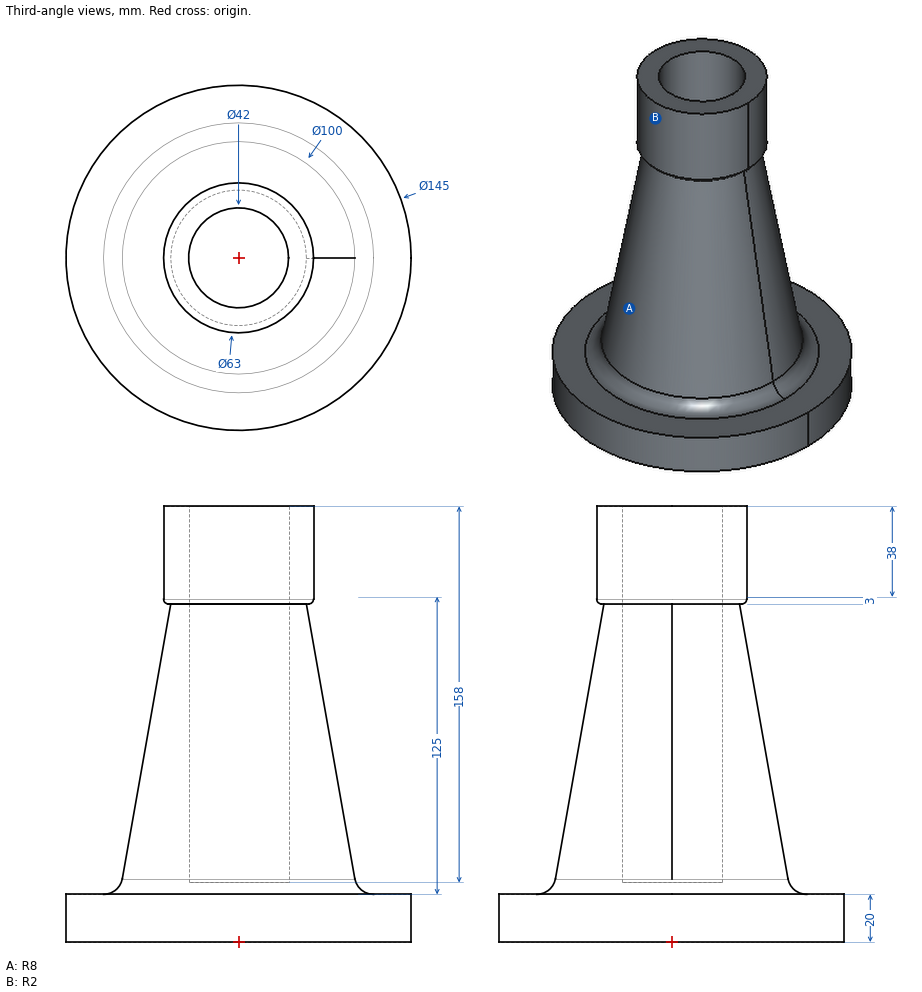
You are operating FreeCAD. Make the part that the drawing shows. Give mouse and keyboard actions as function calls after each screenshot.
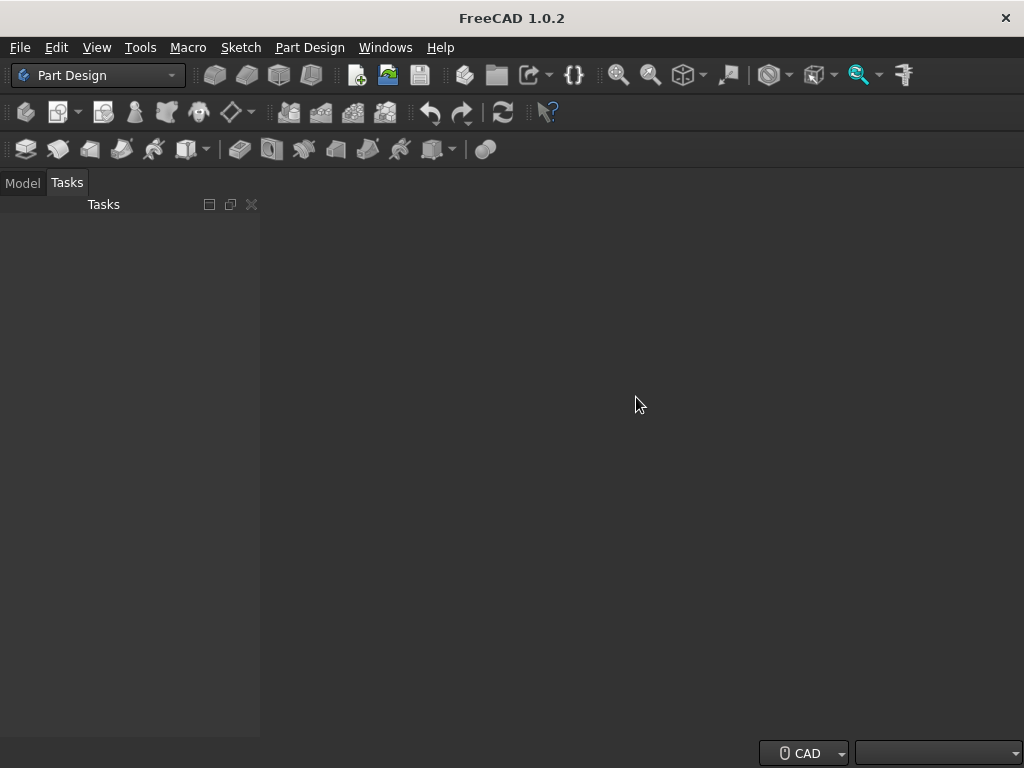
click(356, 76)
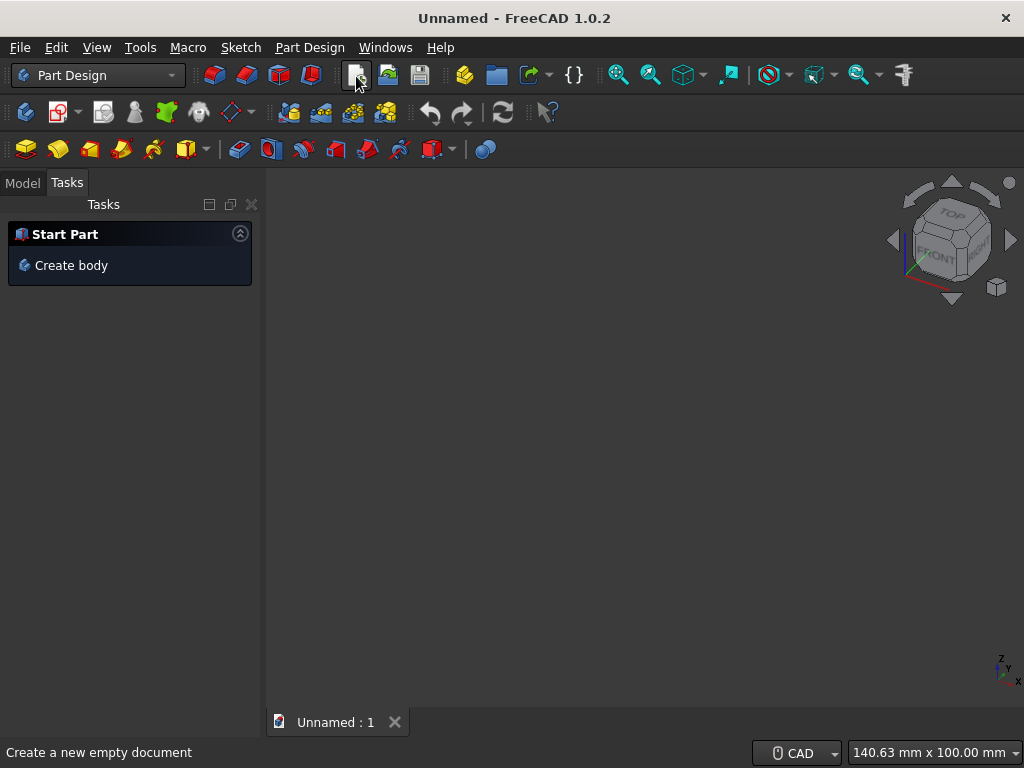
click(58, 112)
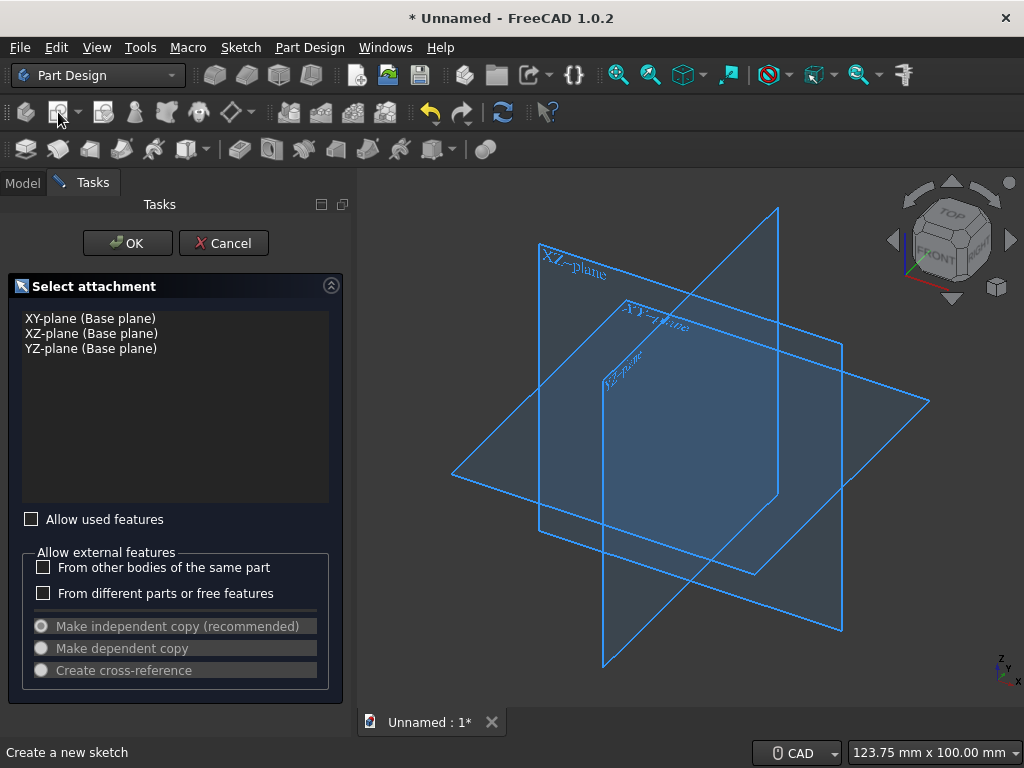
click(82, 318)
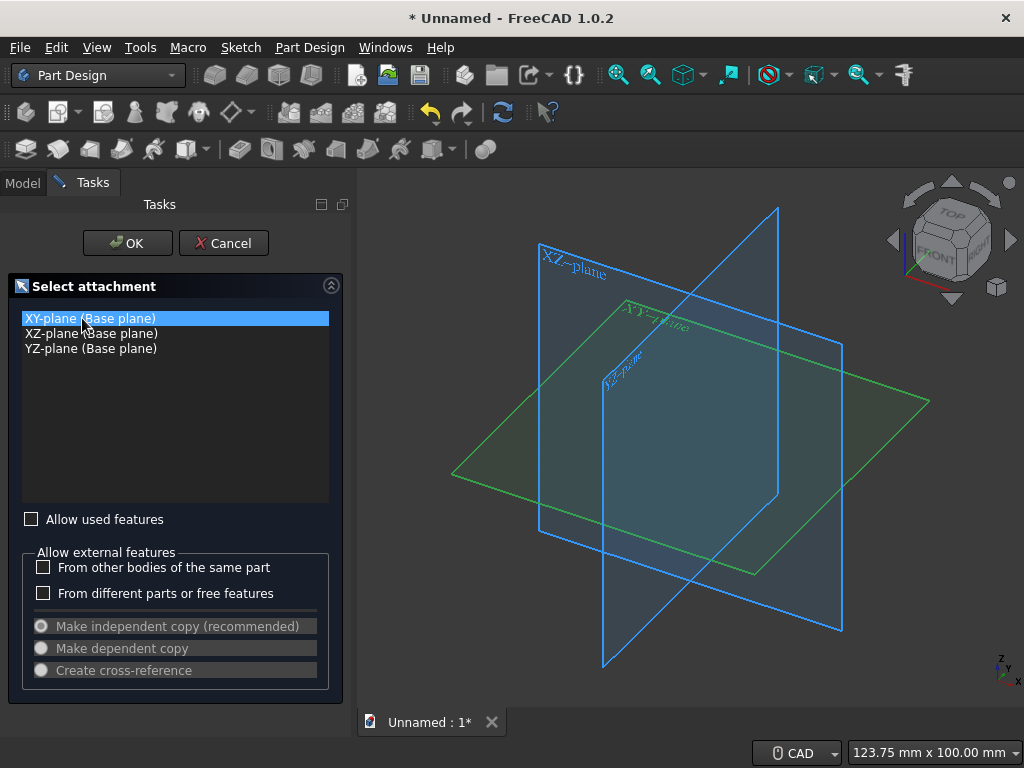
click(128, 243)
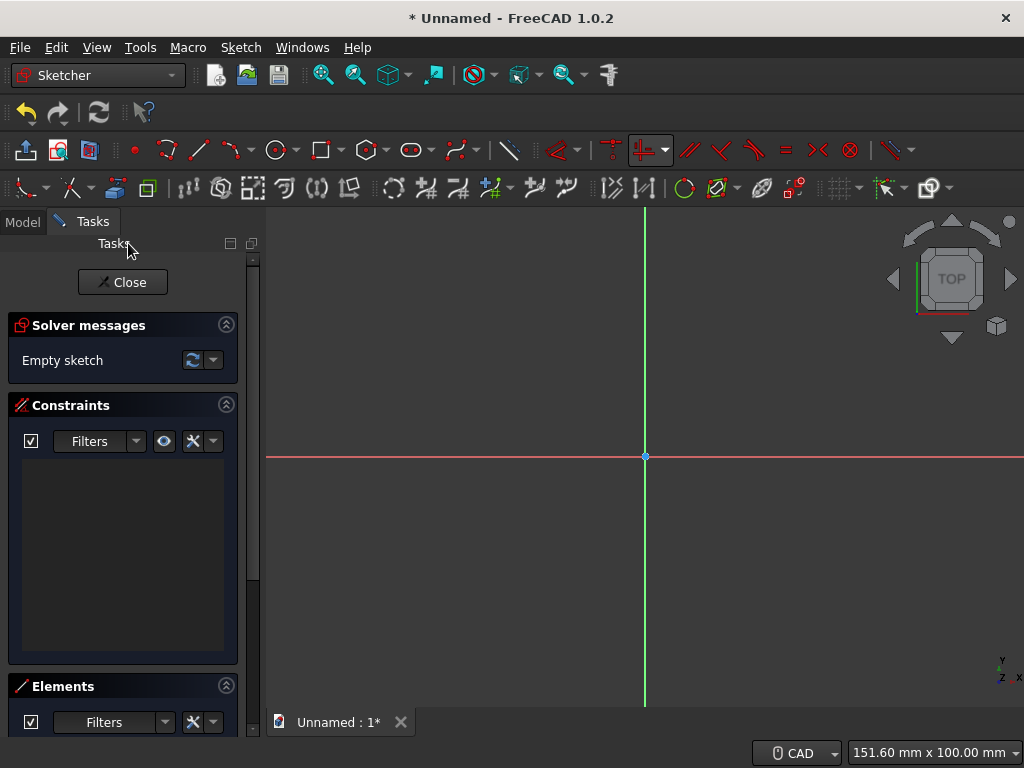
scroll(521, 457, down, 4)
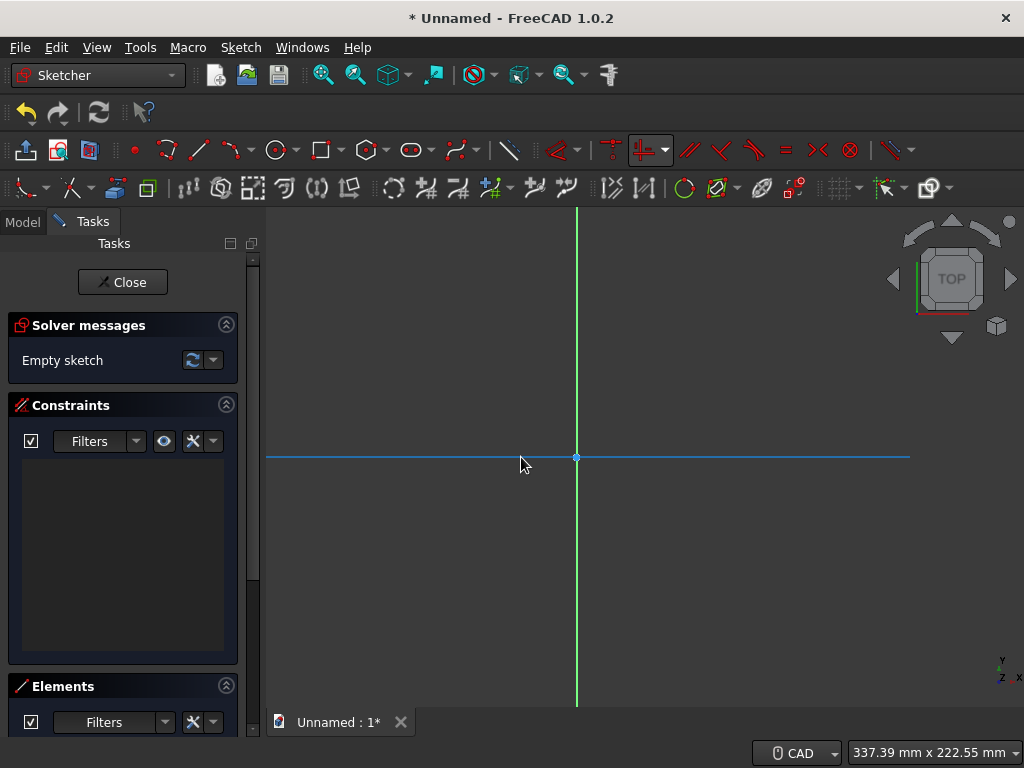
key(g)
key(c)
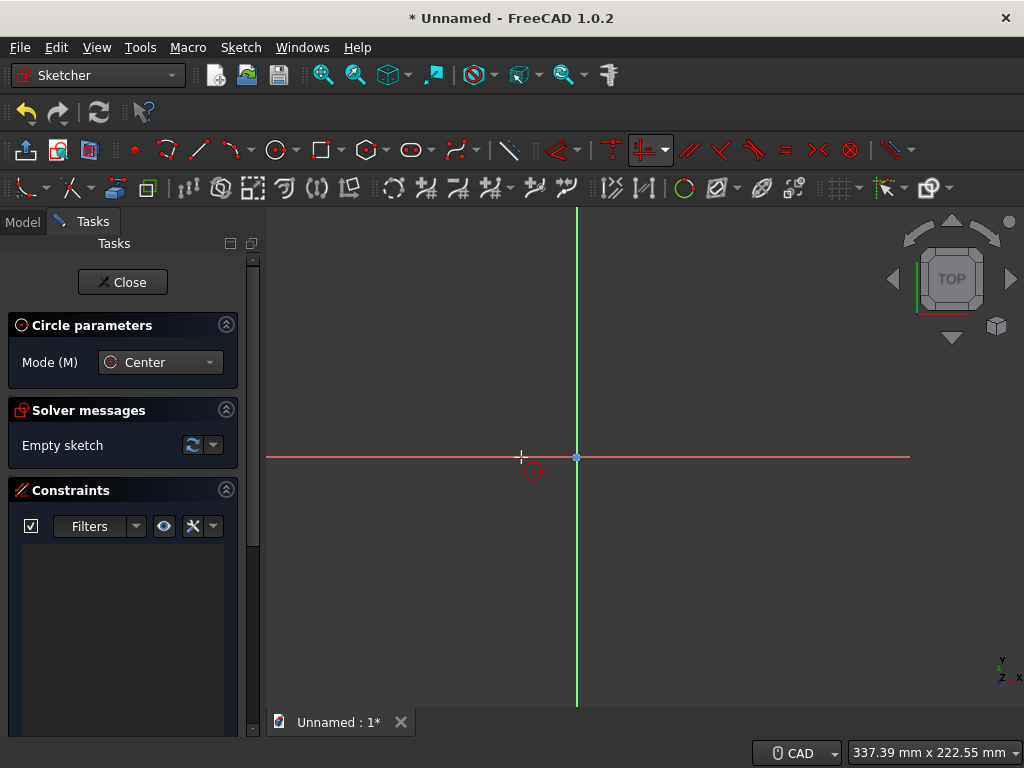
click(577, 457)
click(692, 342)
key(Escape)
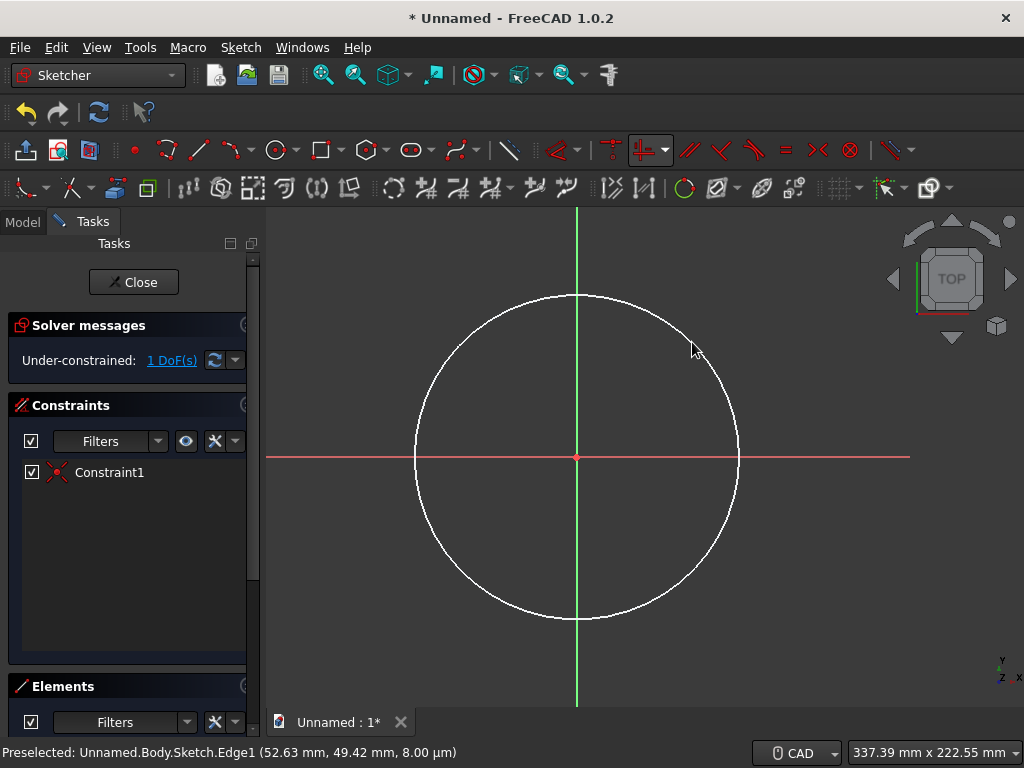
key(d)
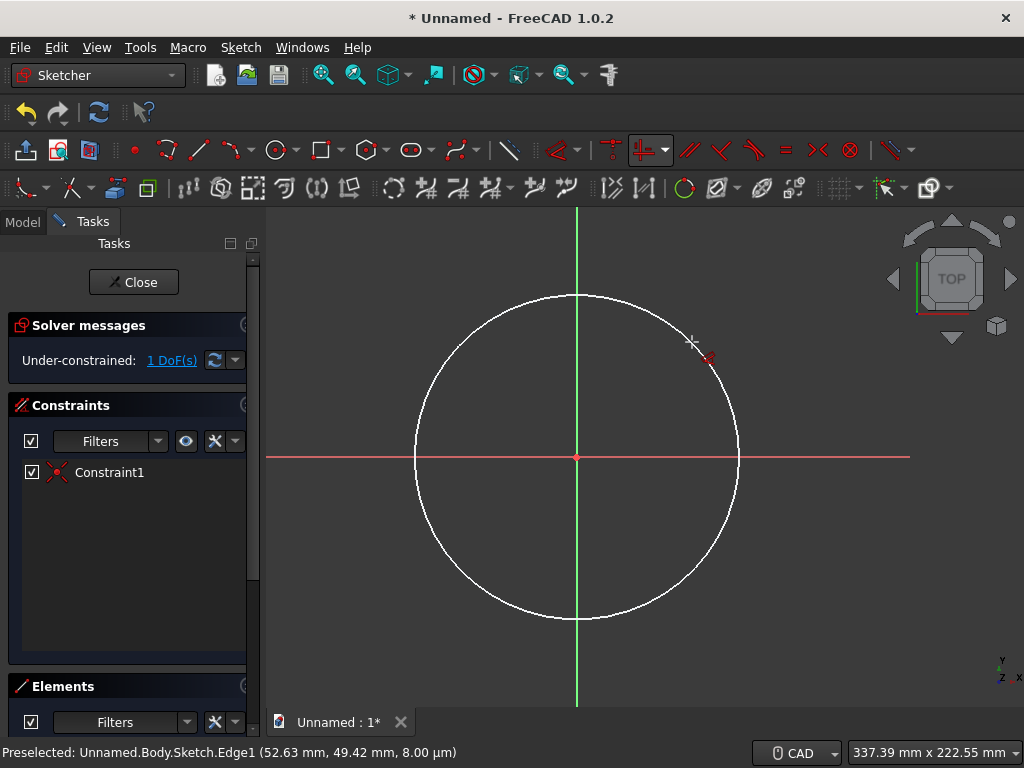
click(691, 342)
click(714, 319)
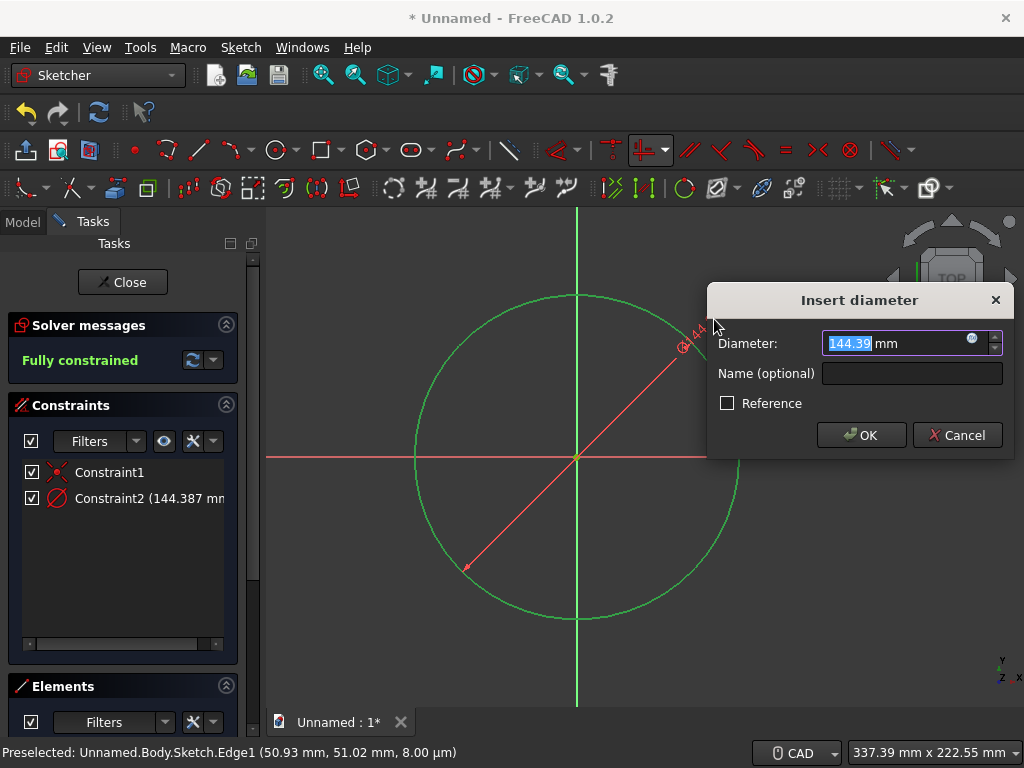
text(145)
key(Return)
key(Escape)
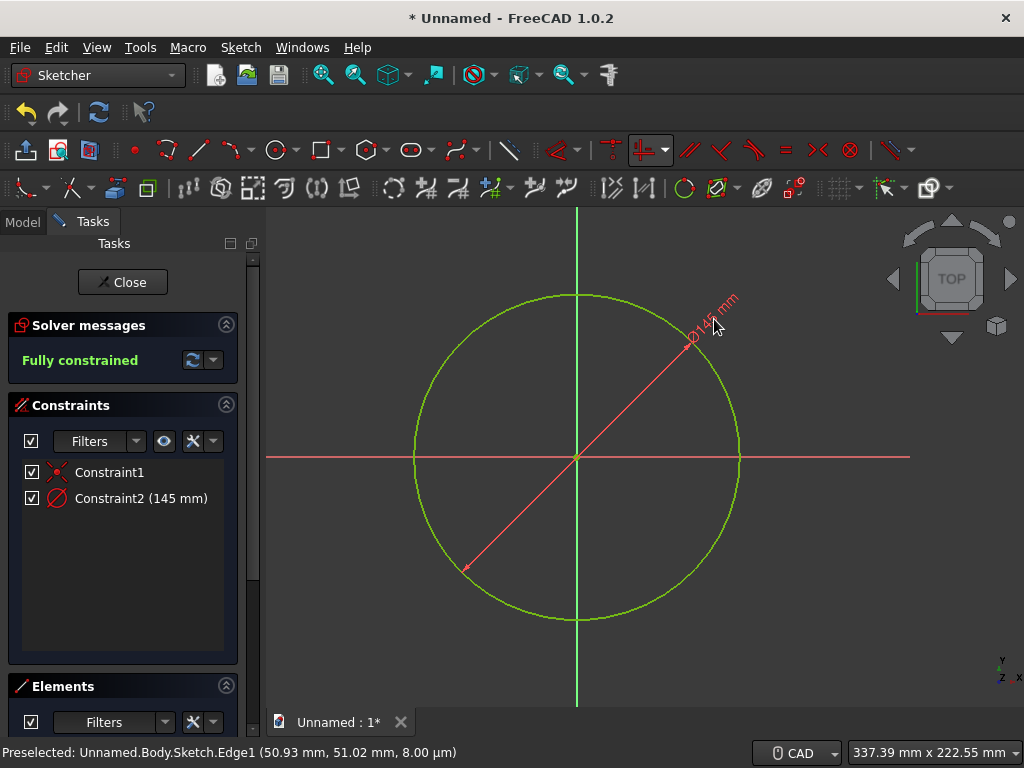
click(123, 282)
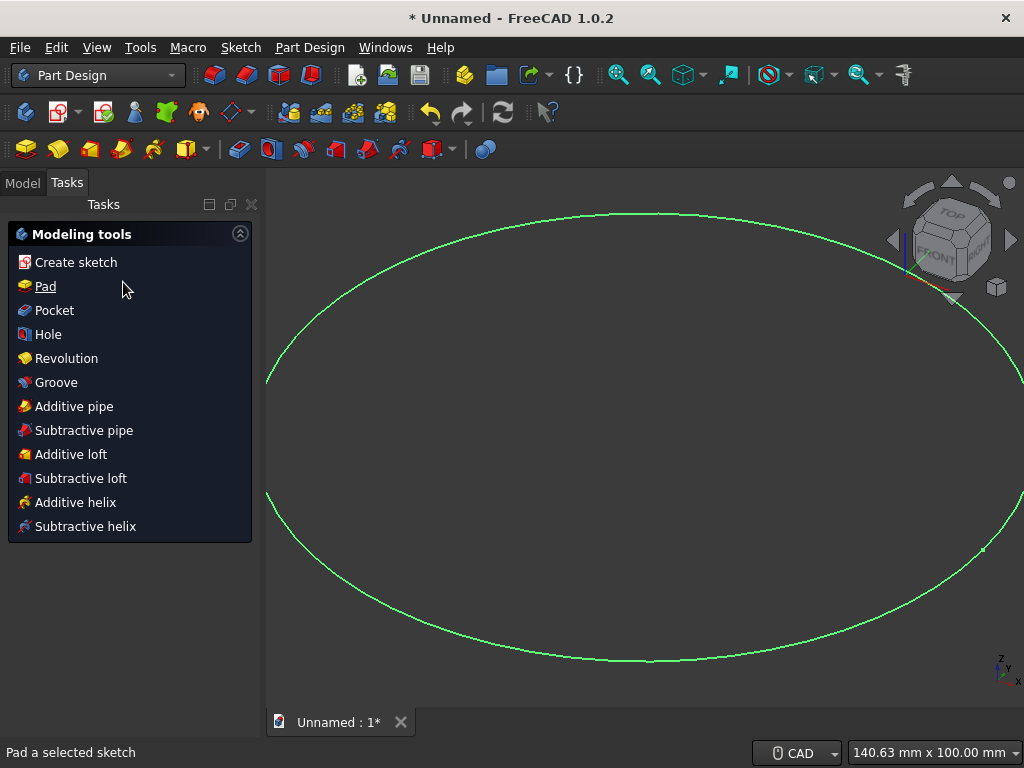
click(26, 150)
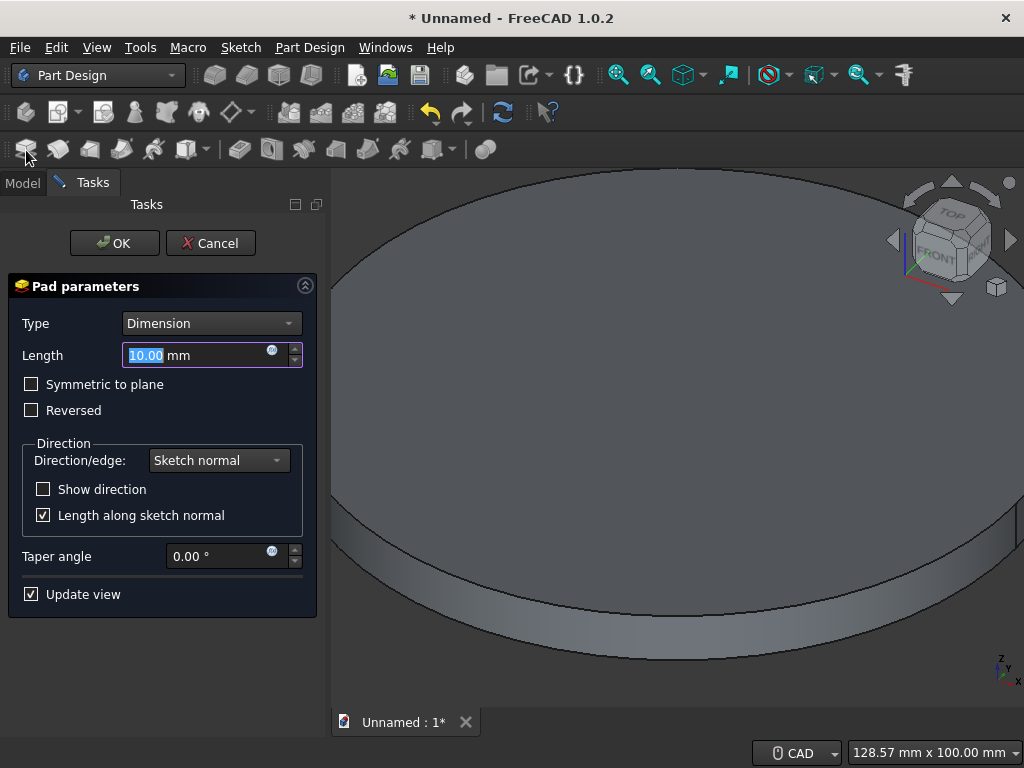
text(20)
key(Tab)